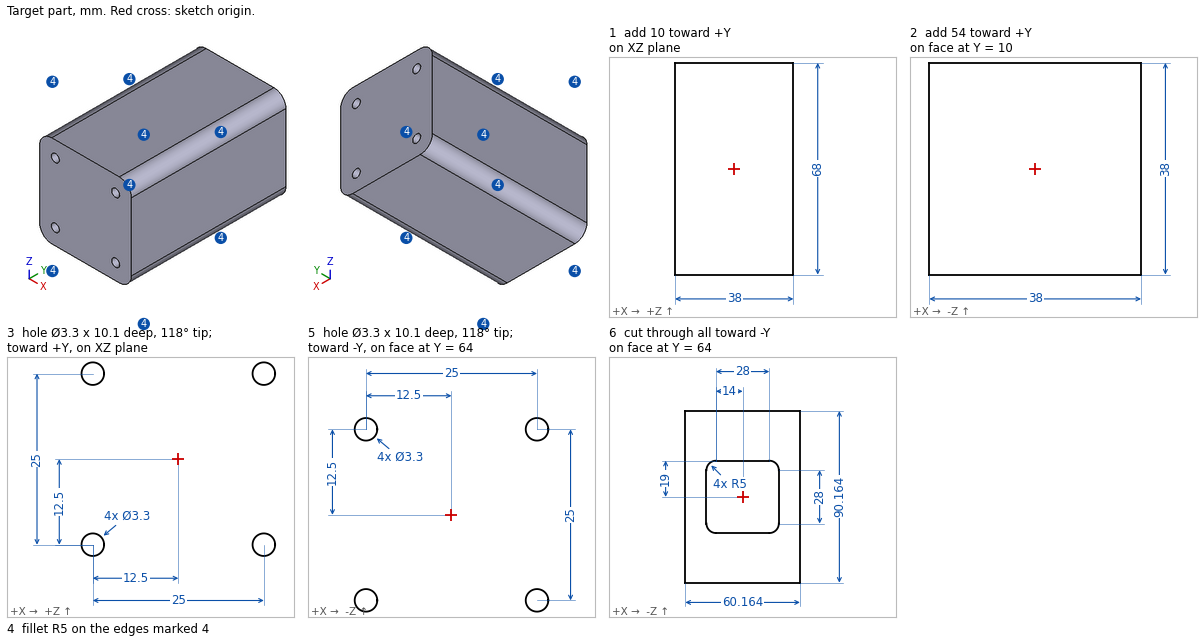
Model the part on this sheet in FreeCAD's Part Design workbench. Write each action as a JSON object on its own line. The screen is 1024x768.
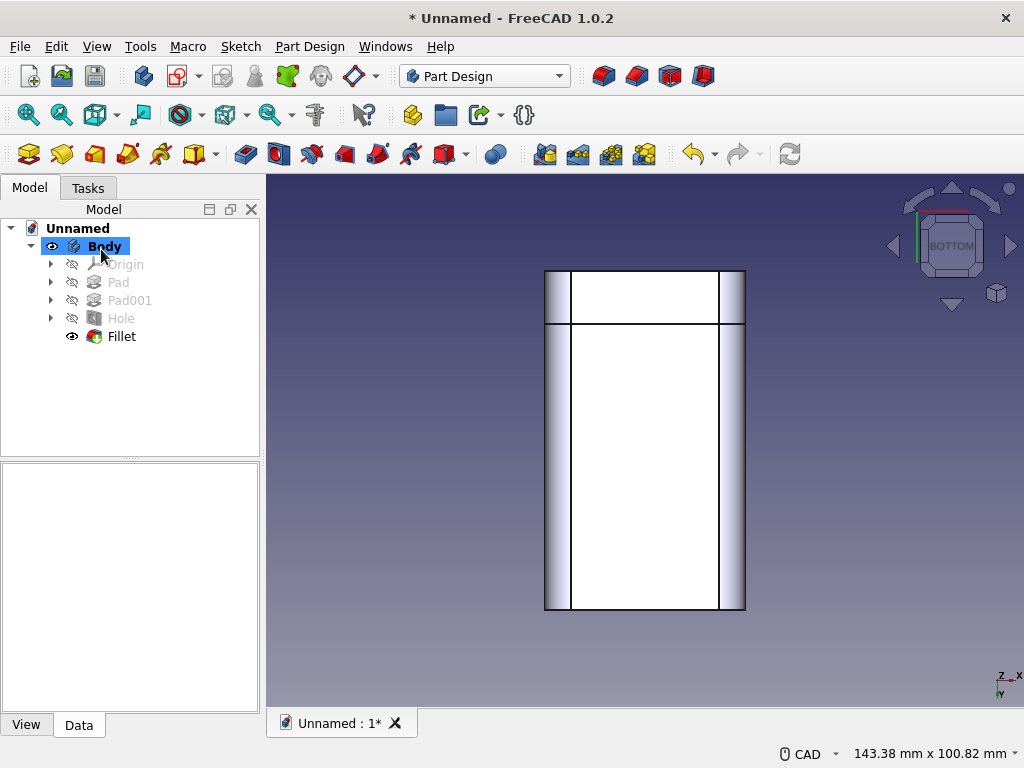
{"action": "key", "text": "4"}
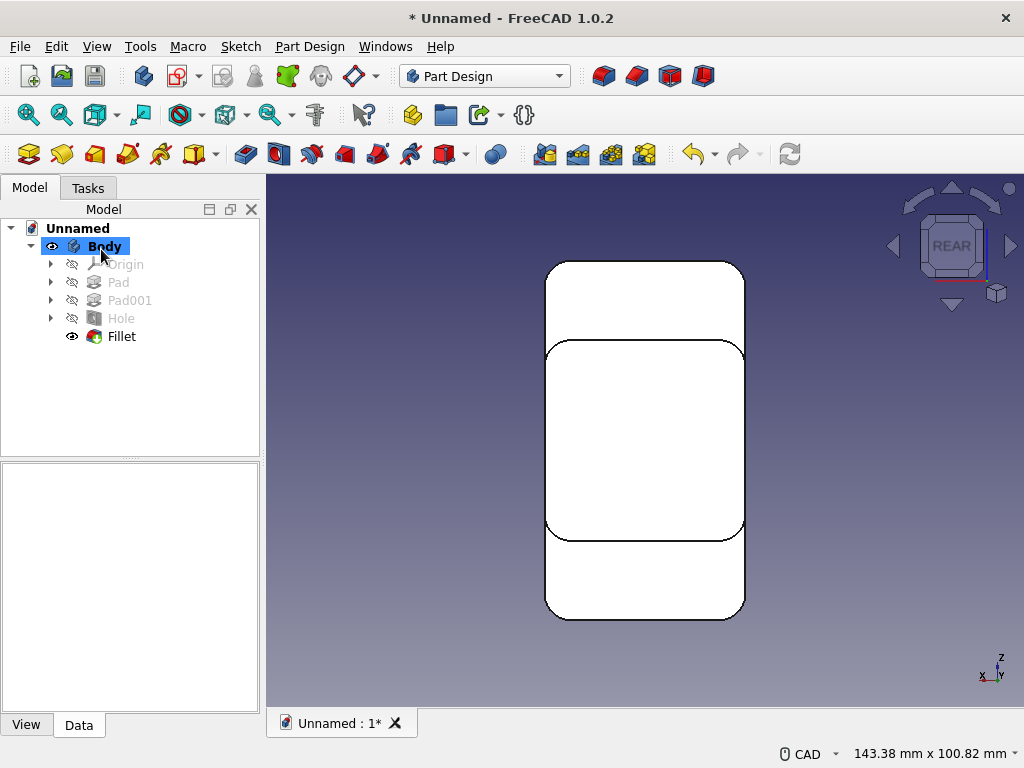
{"action": "left_click", "coordinate": [645, 440]}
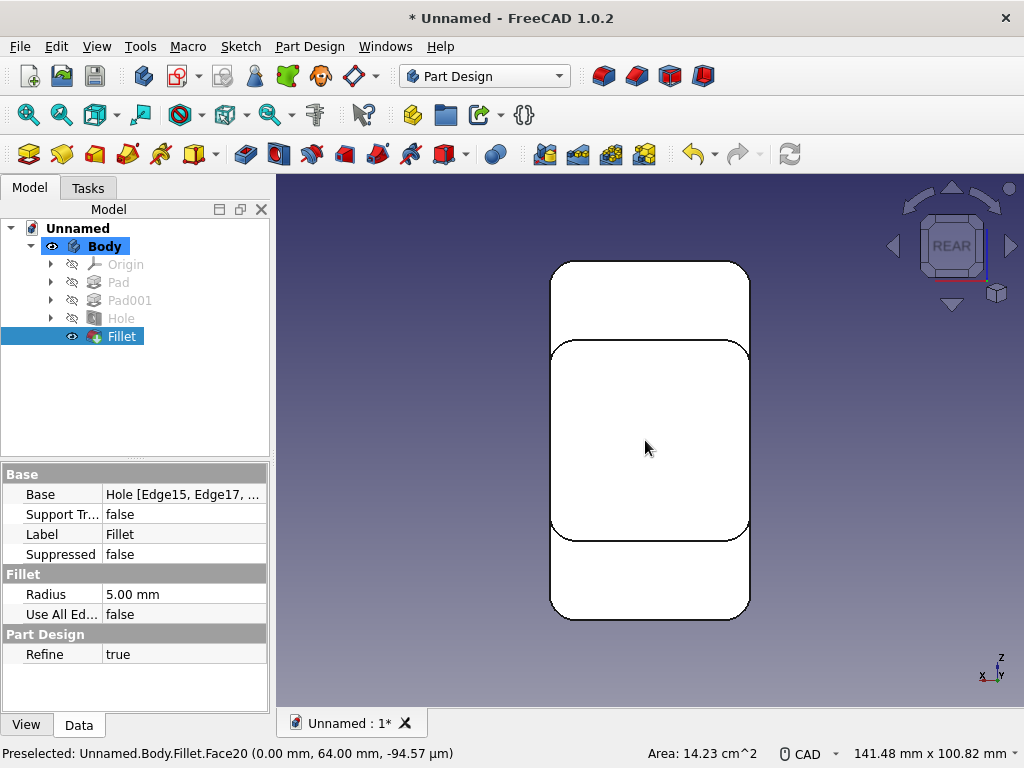
{"action": "left_click", "coordinate": [176, 76]}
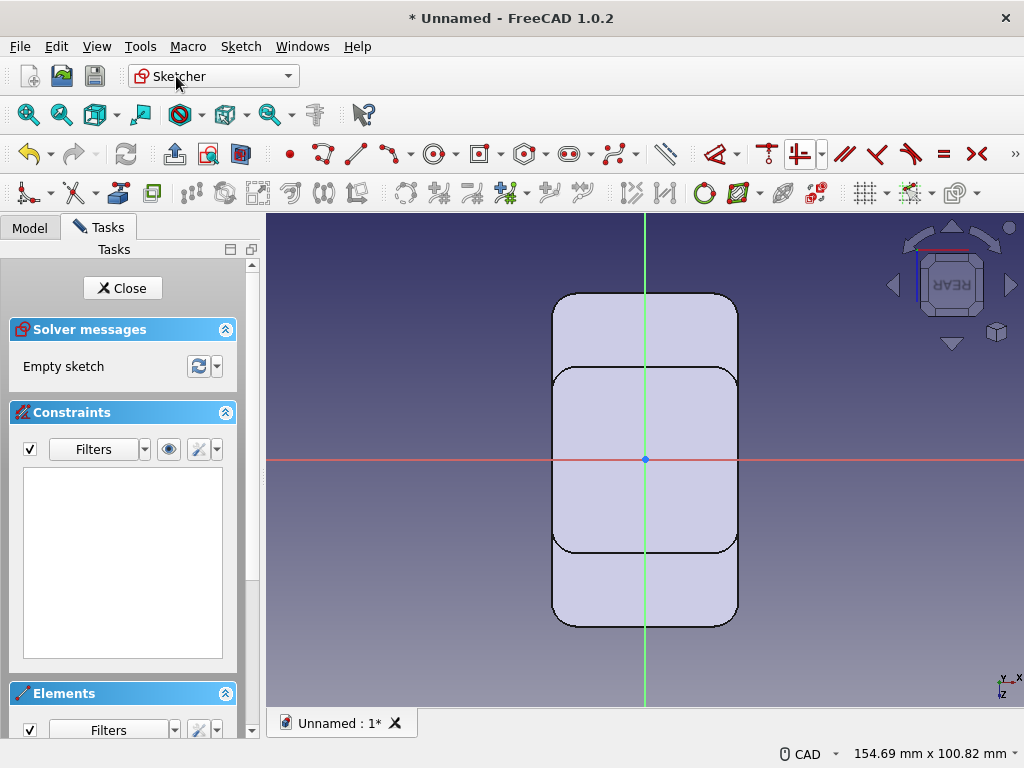
{"action": "scroll", "coordinate": [701, 460], "scroll_direction": "up", "scroll_amount": 4}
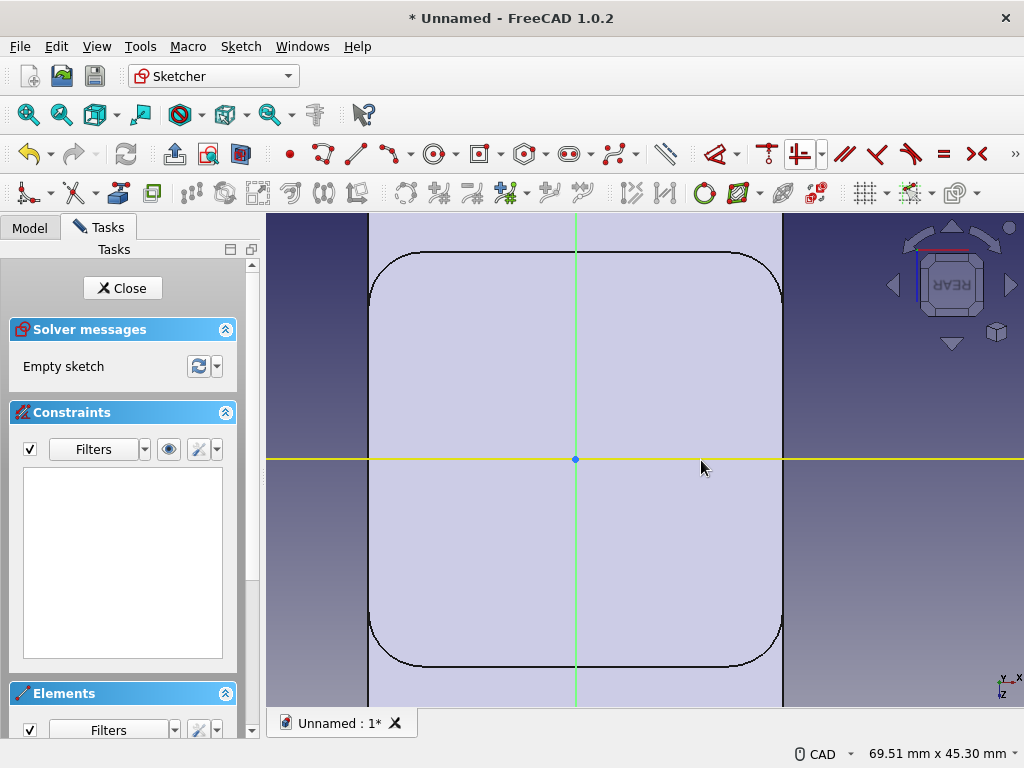
{"action": "left_click", "coordinate": [434, 154]}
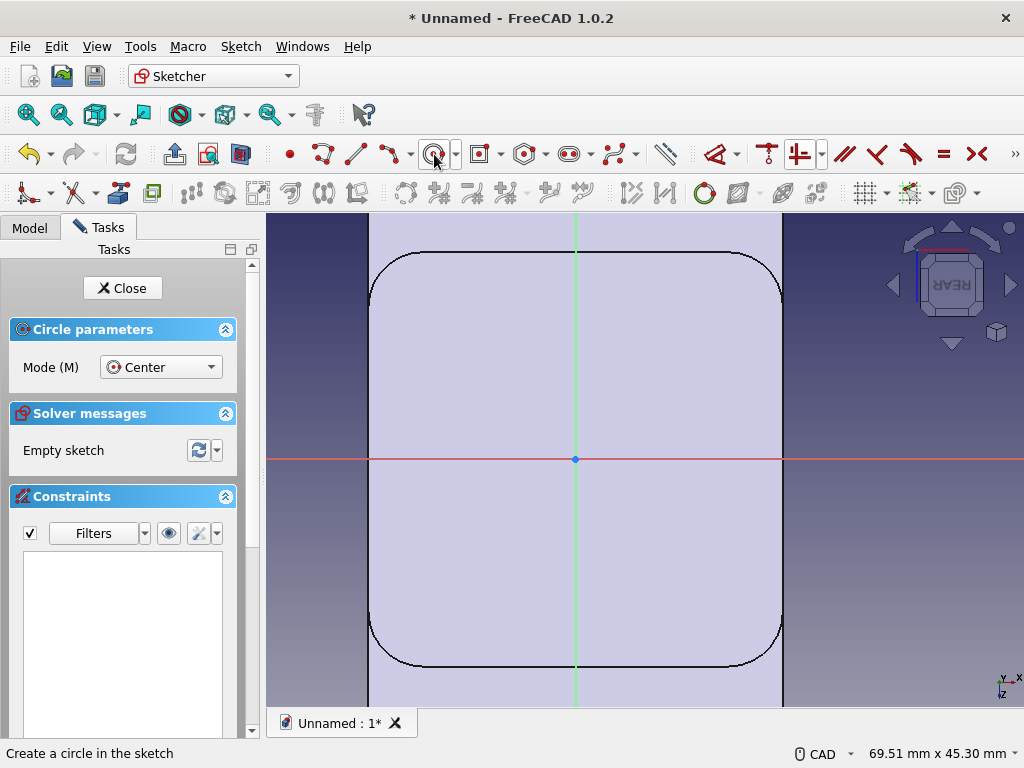
{"action": "scroll", "coordinate": [439, 323], "scroll_direction": "up", "scroll_amount": 2}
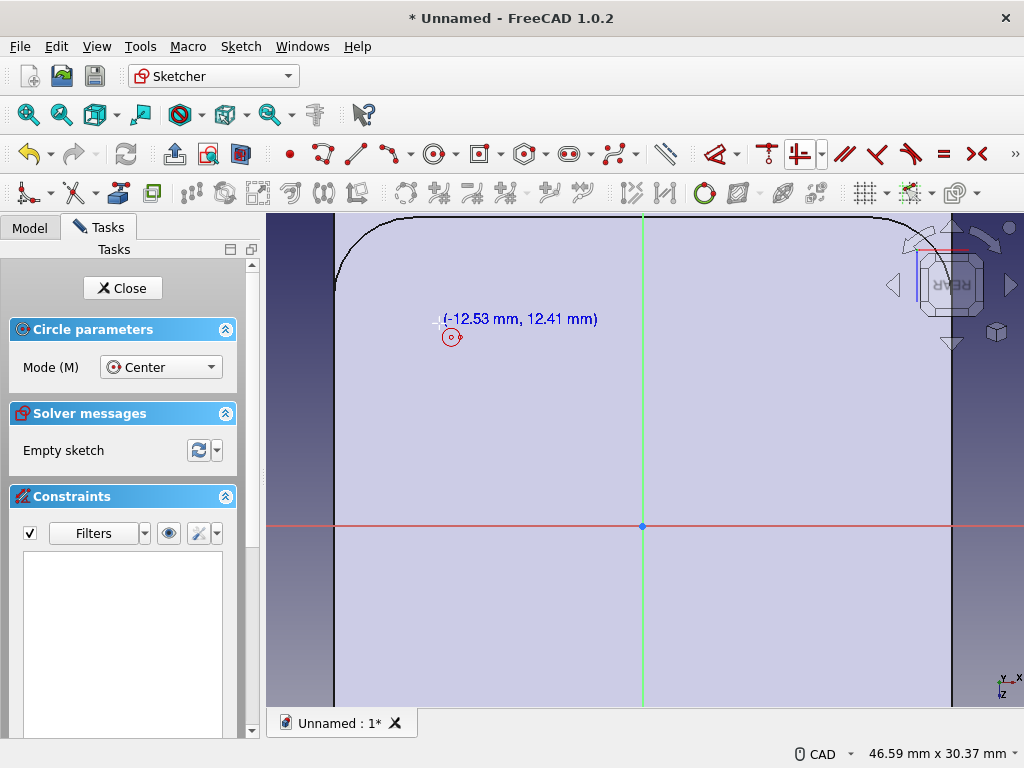
{"action": "left_click", "coordinate": [439, 323]}
{"action": "left_click", "coordinate": [458, 304]}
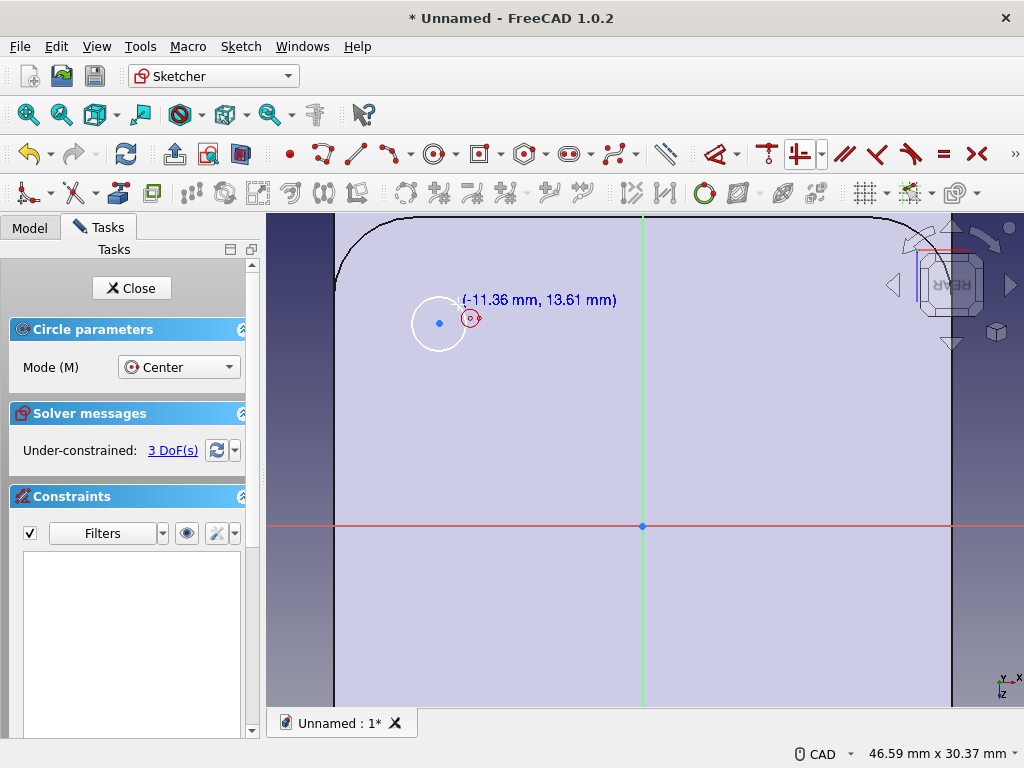
{"action": "left_click", "coordinate": [846, 323]}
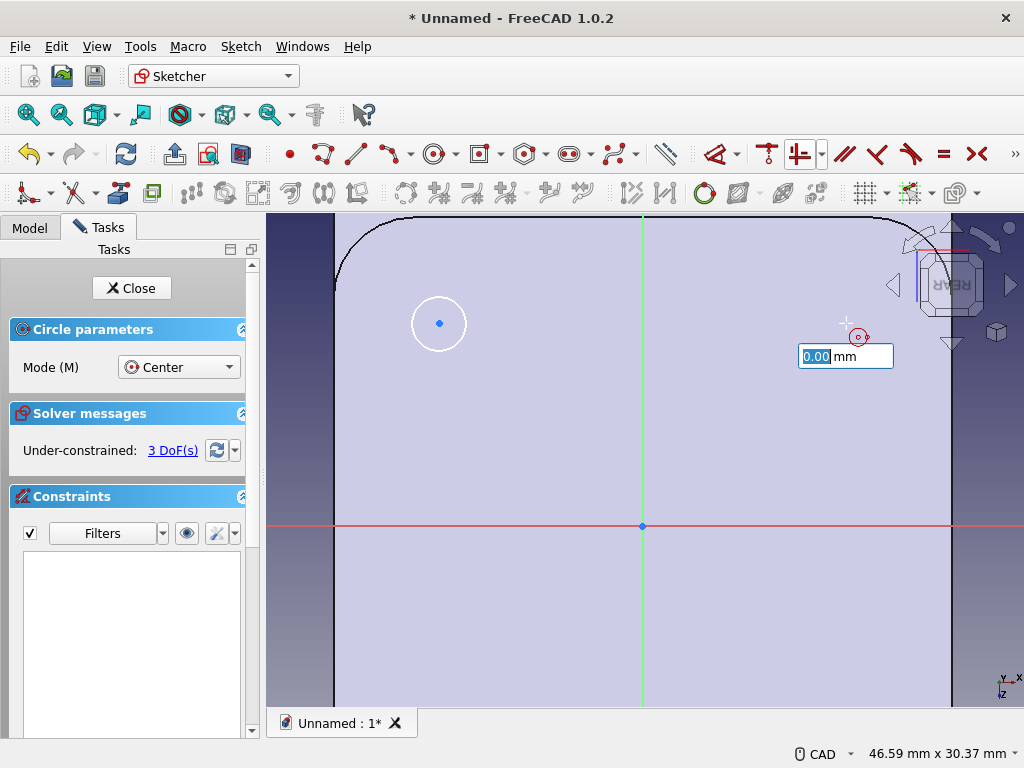
{"action": "scroll", "coordinate": [442, 325], "scroll_direction": "down", "scroll_amount": 2}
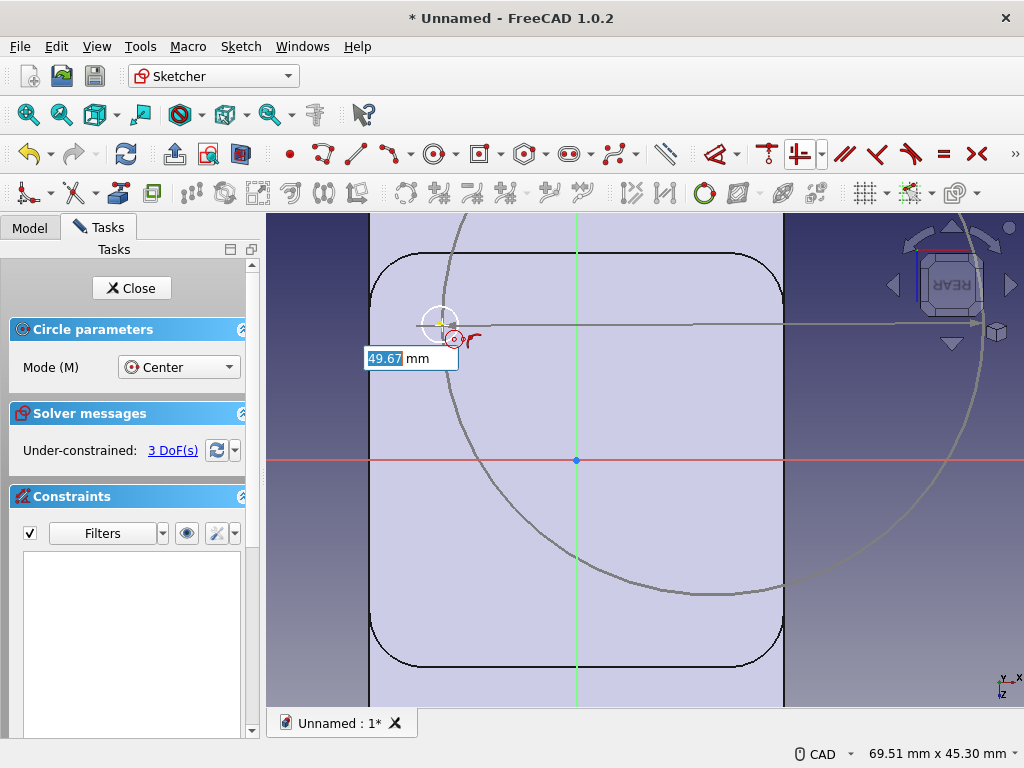
{"action": "left_click", "coordinate": [726, 311]}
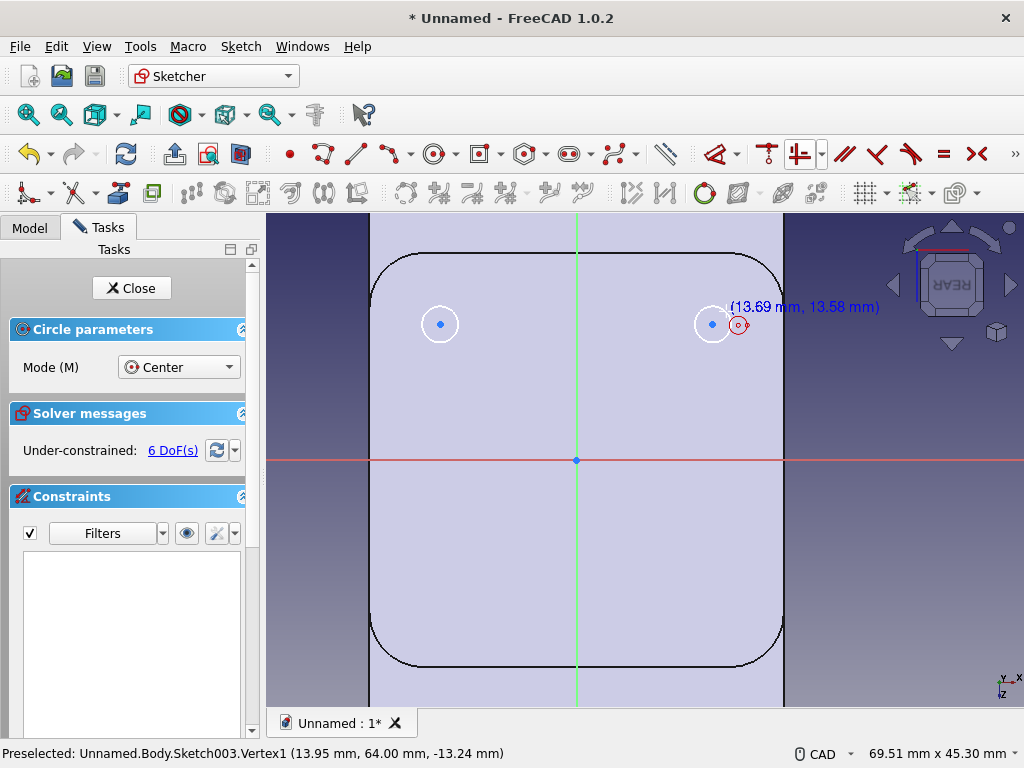
{"action": "scroll", "coordinate": [713, 596], "scroll_direction": "up", "scroll_amount": 2}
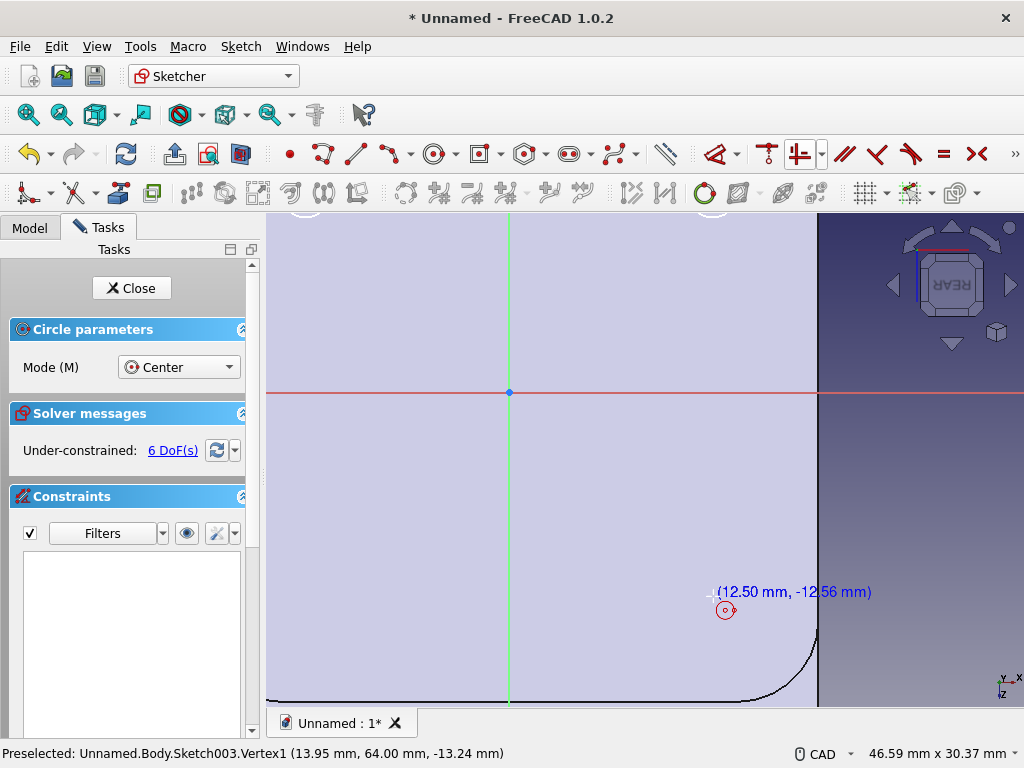
{"action": "left_click", "coordinate": [713, 596]}
{"action": "left_click", "coordinate": [732, 577]}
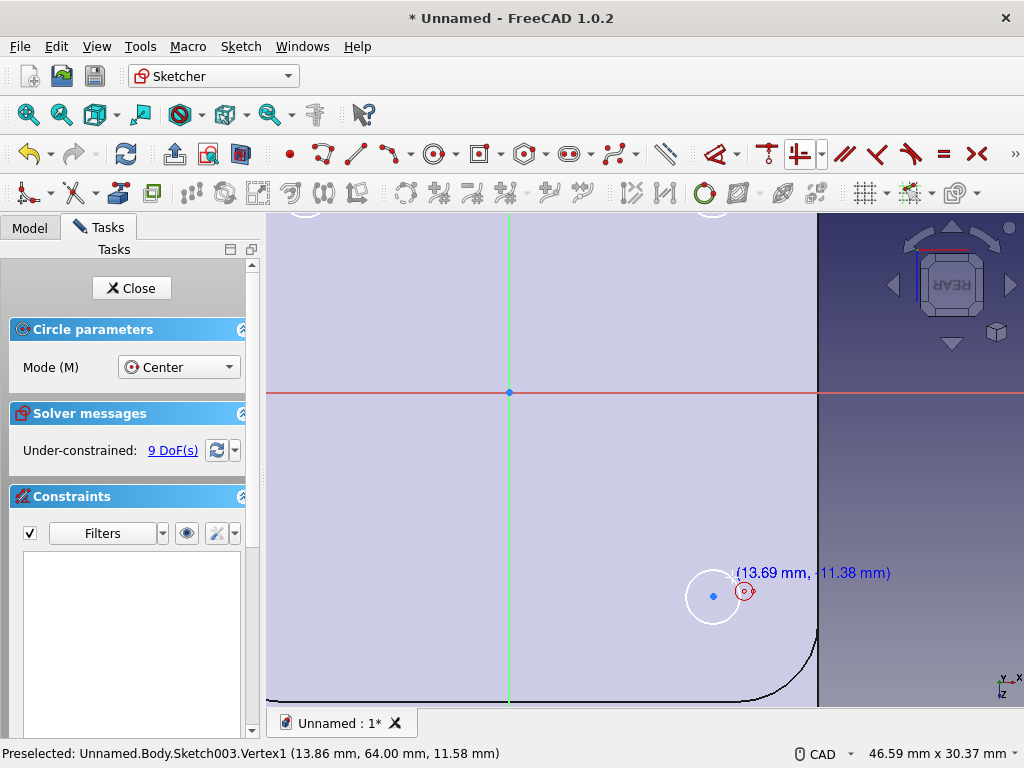
{"action": "left_click", "coordinate": [306, 596]}
{"action": "left_click", "coordinate": [325, 577]}
{"action": "key", "text": "Escape"}